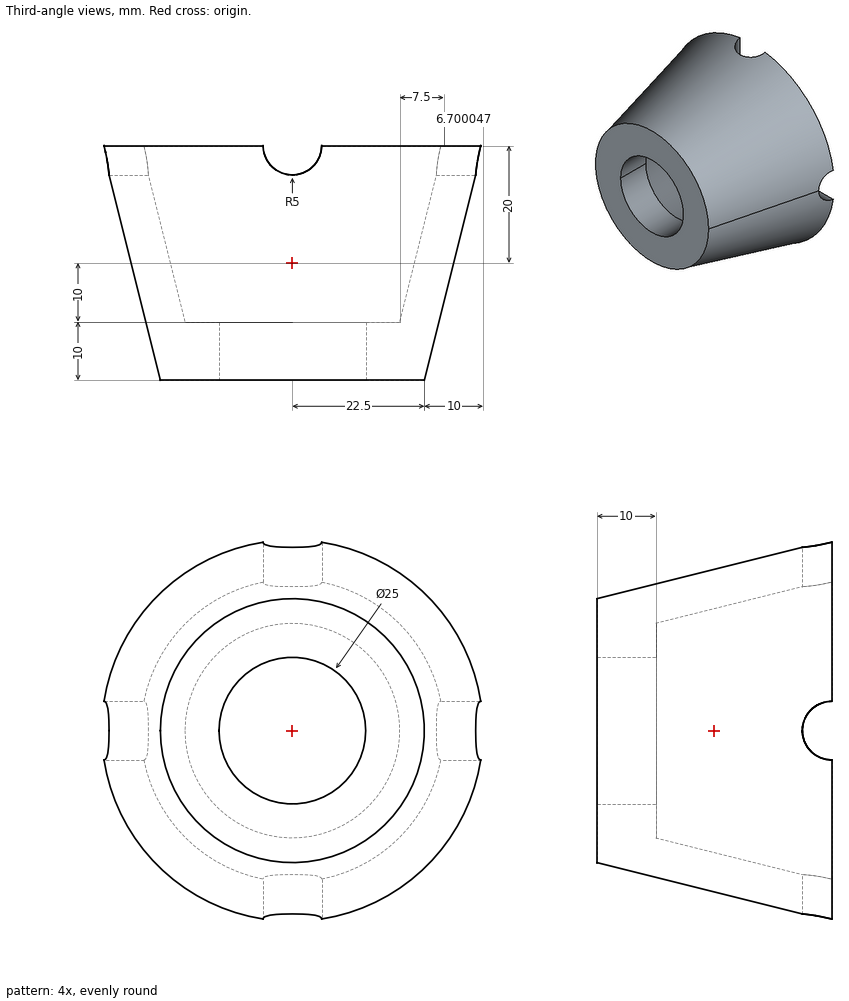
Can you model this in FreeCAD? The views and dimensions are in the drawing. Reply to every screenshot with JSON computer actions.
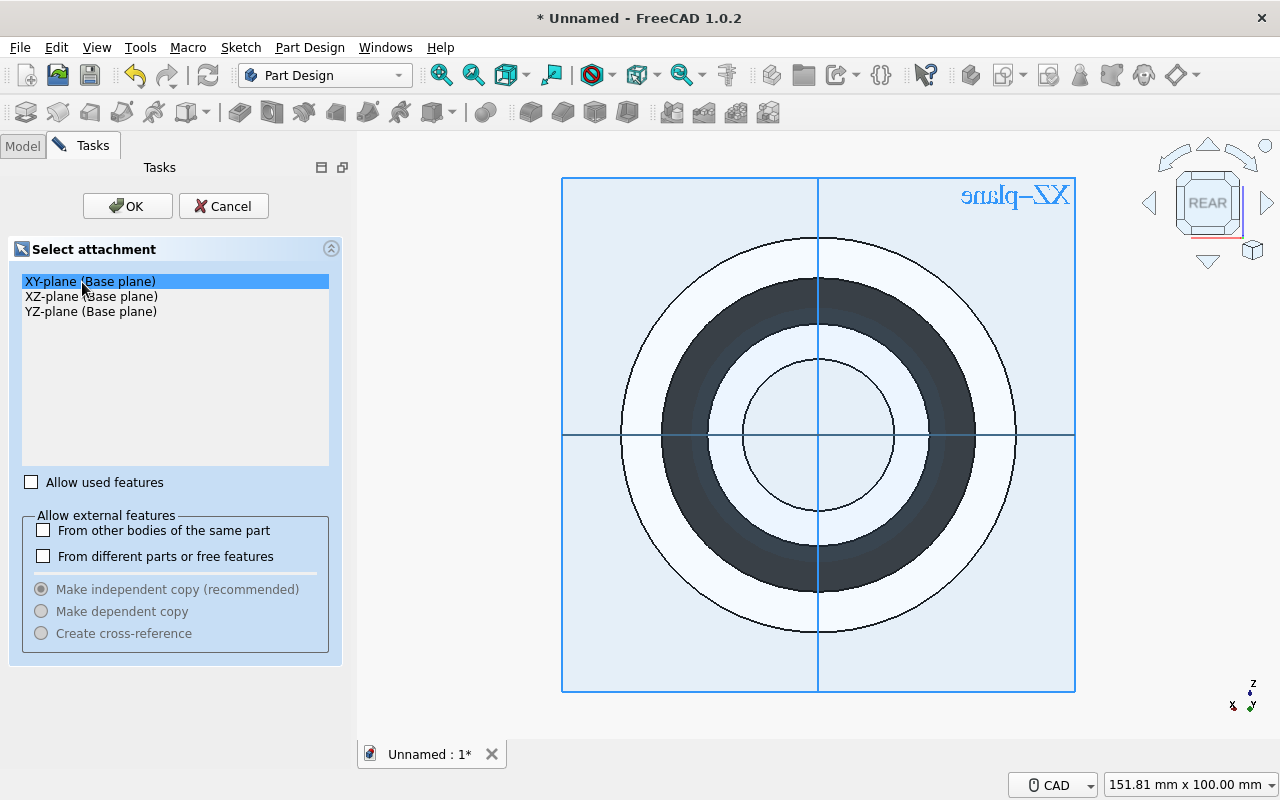
{"action": "left_click", "coordinate": [128, 206]}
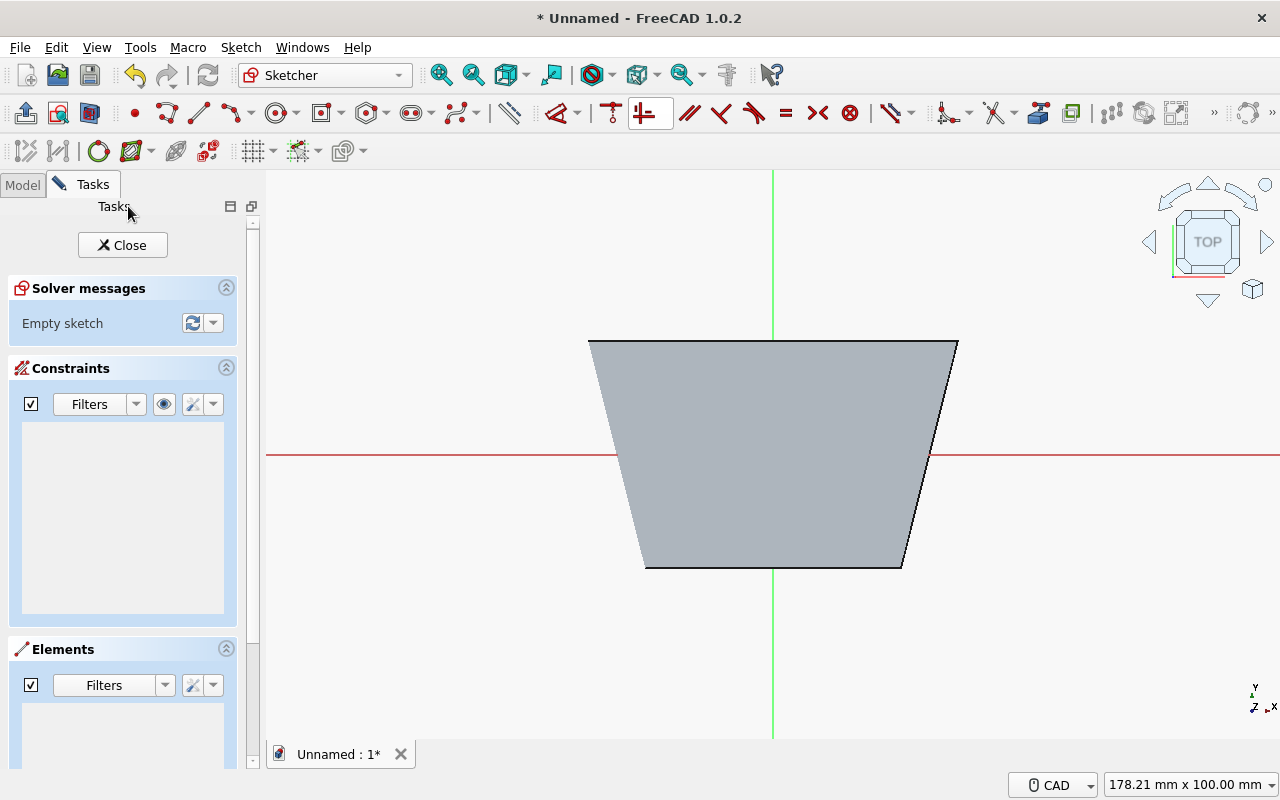
{"action": "left_click", "coordinate": [90, 114]}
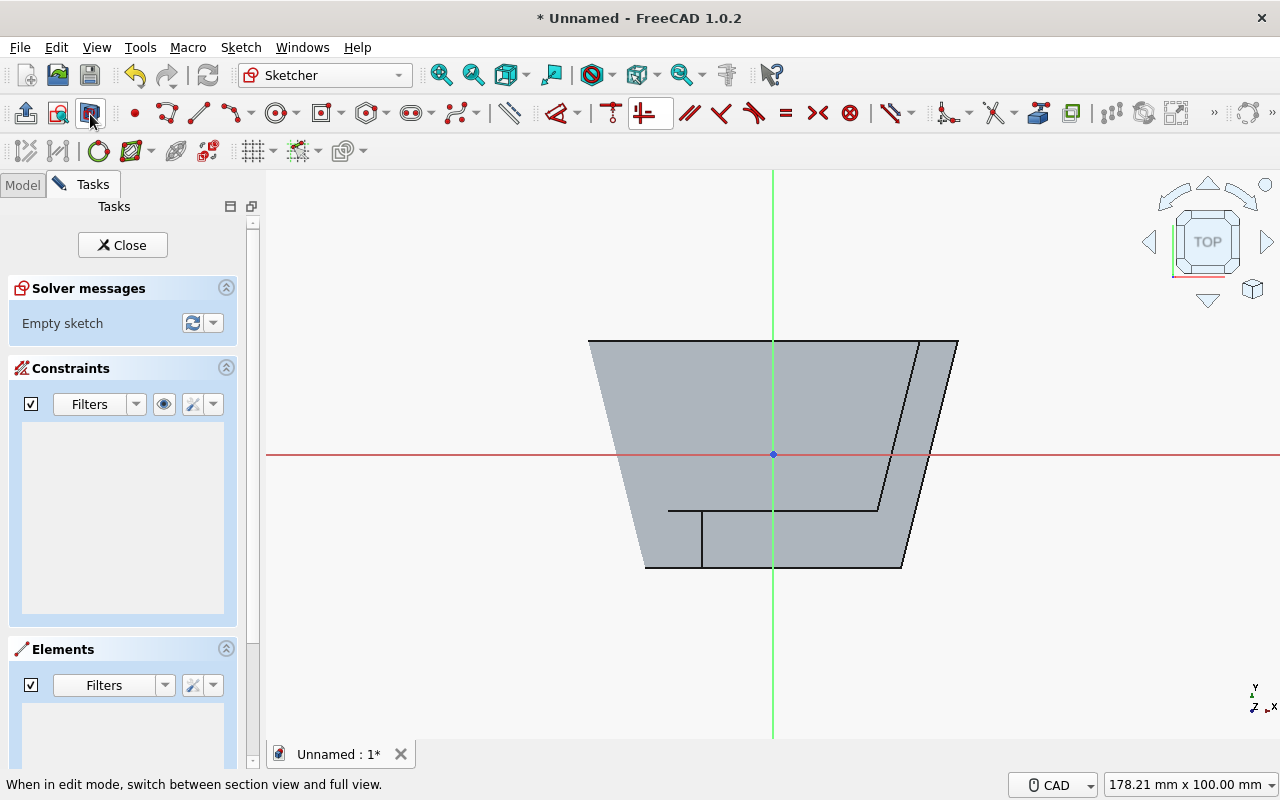
{"action": "scroll", "coordinate": [803, 373], "scroll_direction": "up", "scroll_amount": 6}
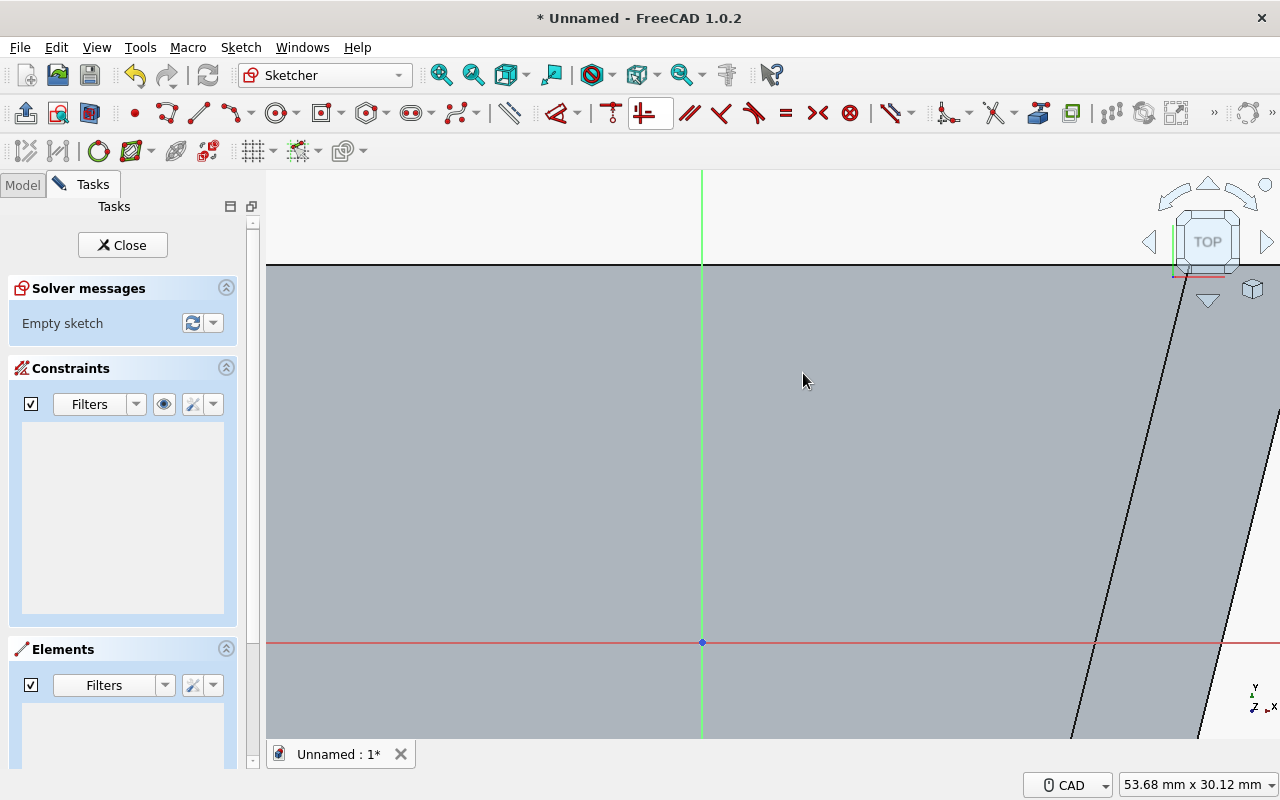
{"action": "left_click", "coordinate": [200, 114]}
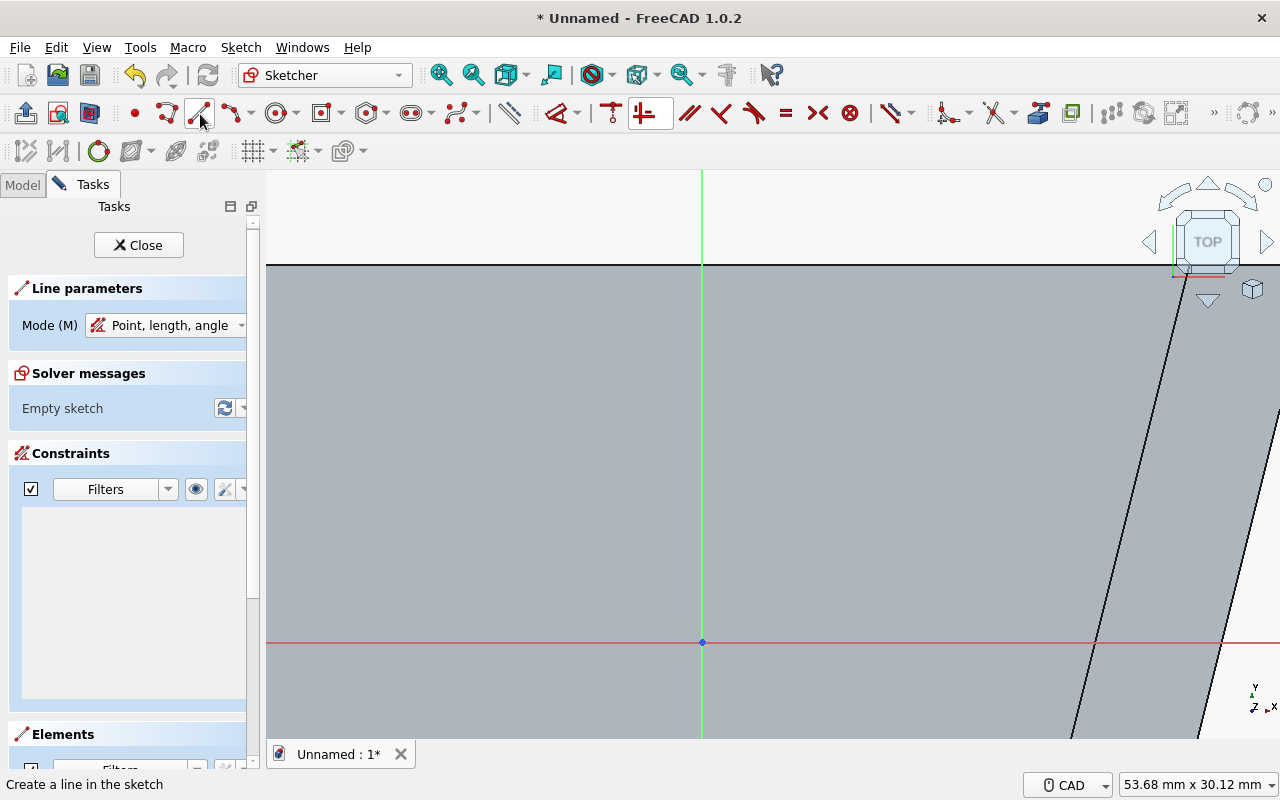
{"action": "left_click", "coordinate": [797, 265]}
{"action": "left_click", "coordinate": [608, 265]}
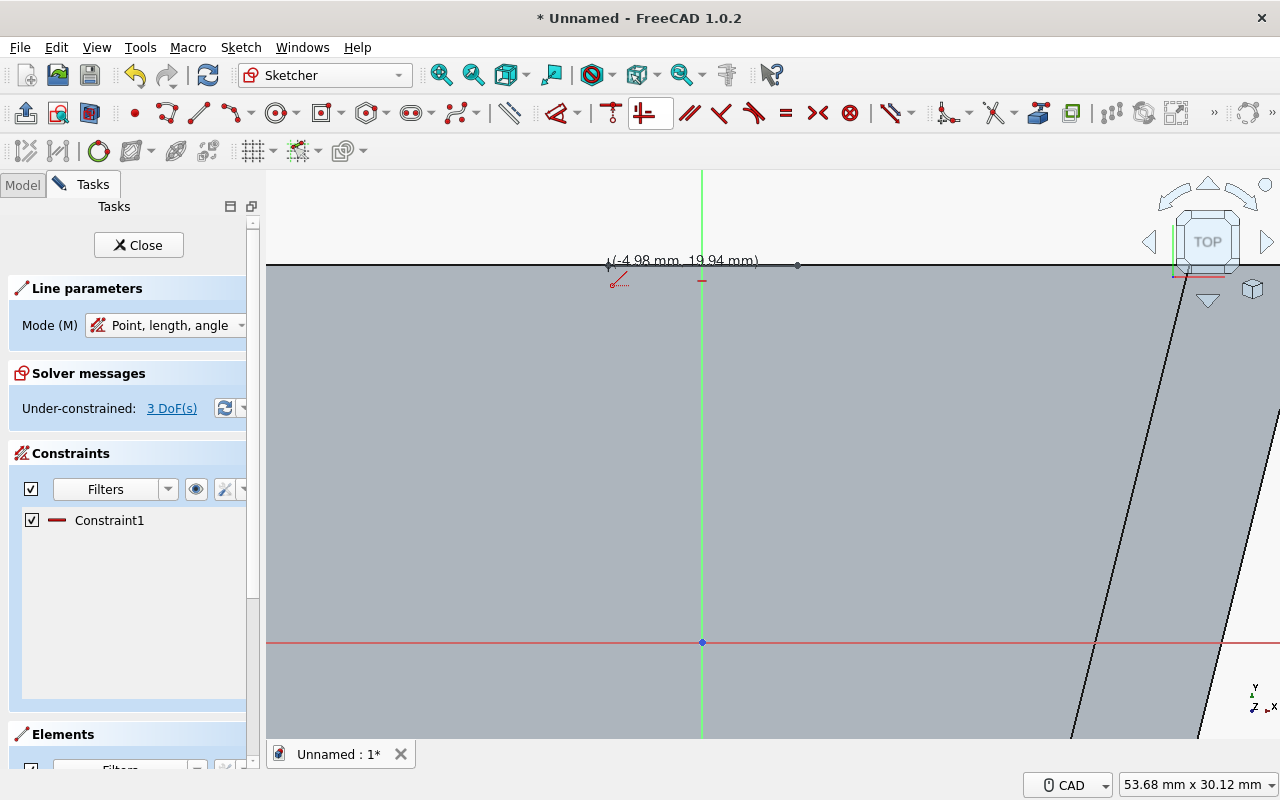
{"action": "left_click", "coordinate": [232, 114]}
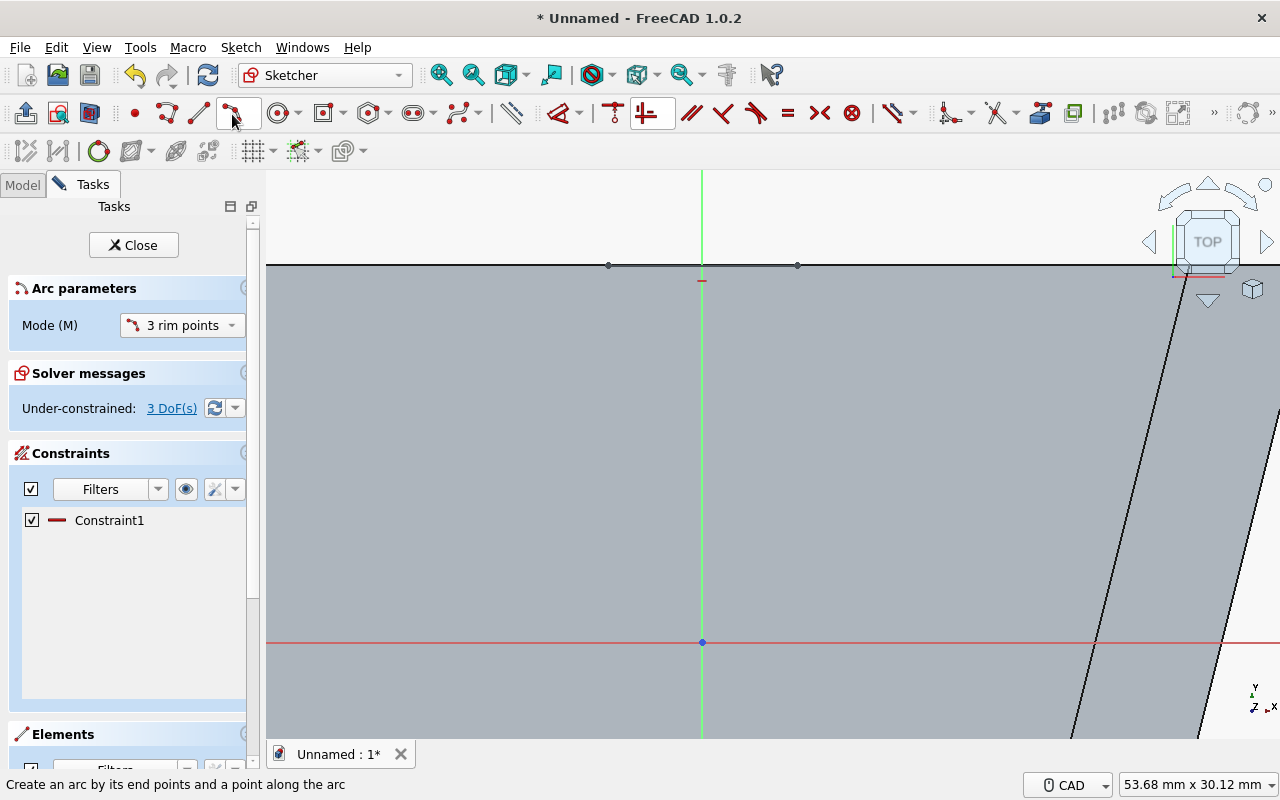
{"action": "left_click", "coordinate": [608, 266]}
{"action": "left_click", "coordinate": [797, 266]}
{"action": "left_click", "coordinate": [673, 355]}
{"action": "key", "text": "Escape"}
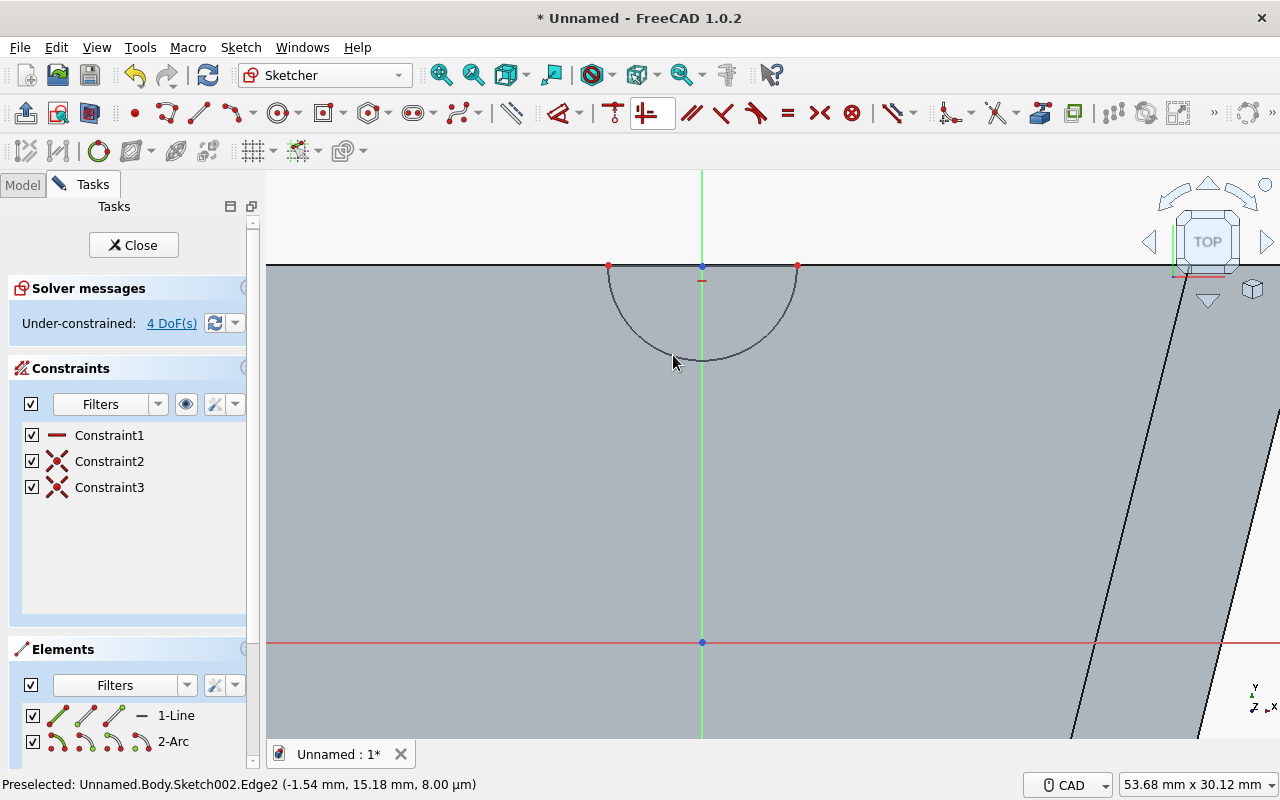
{"action": "left_click", "coordinate": [703, 266]}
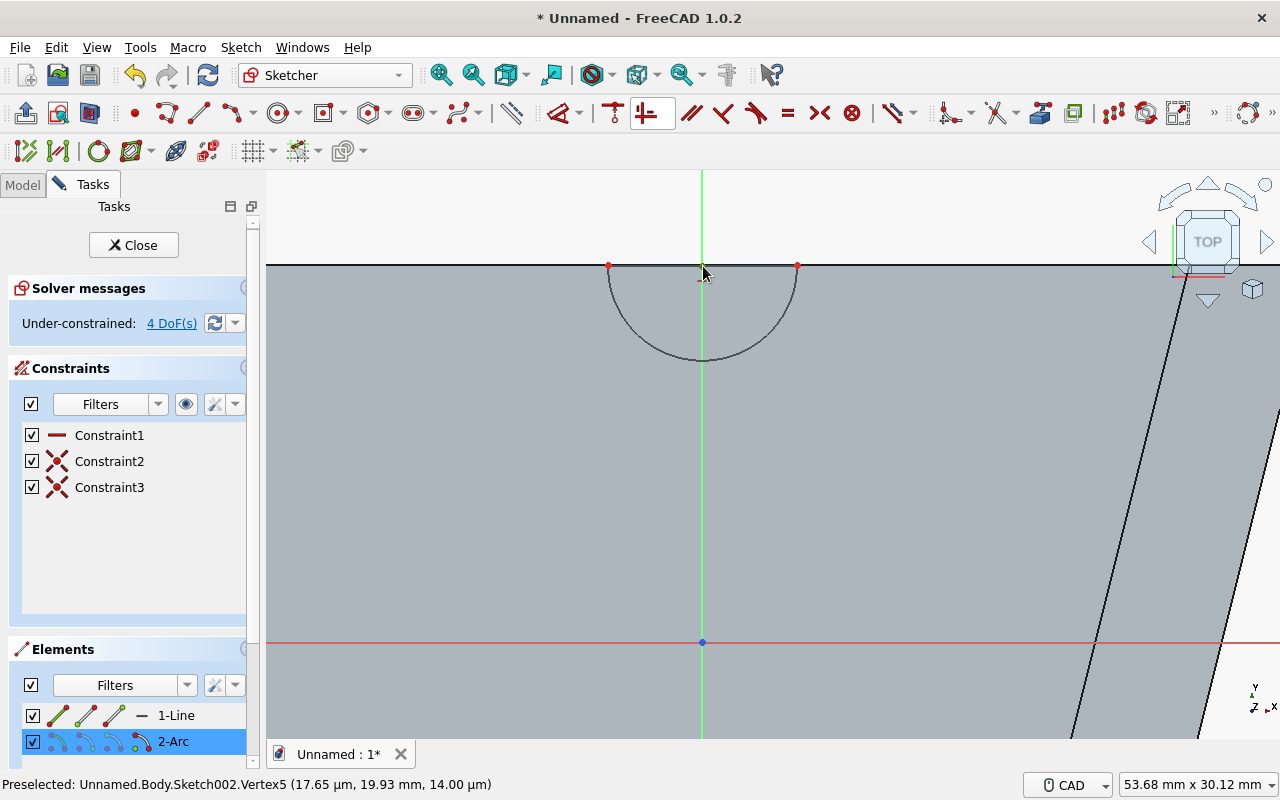
{"action": "left_click", "coordinate": [702, 674]}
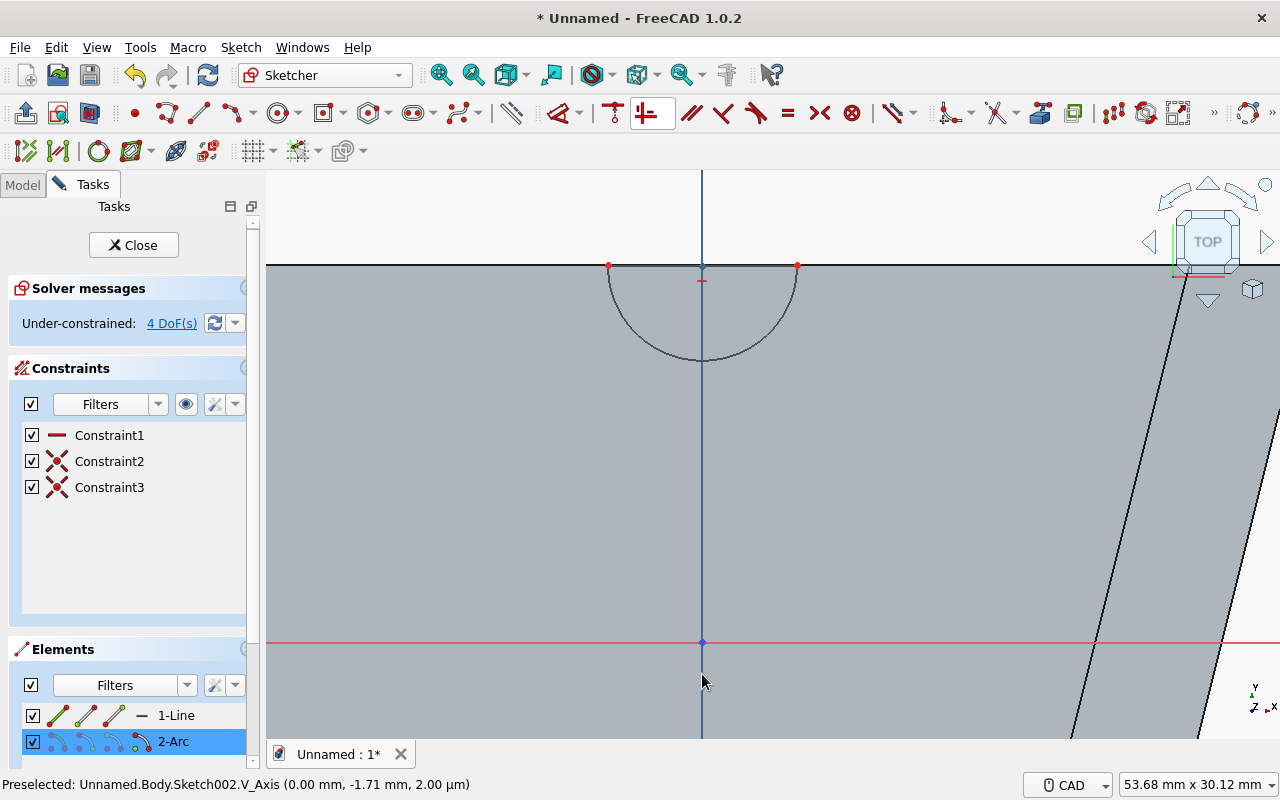
{"action": "left_click", "coordinate": [614, 114]}